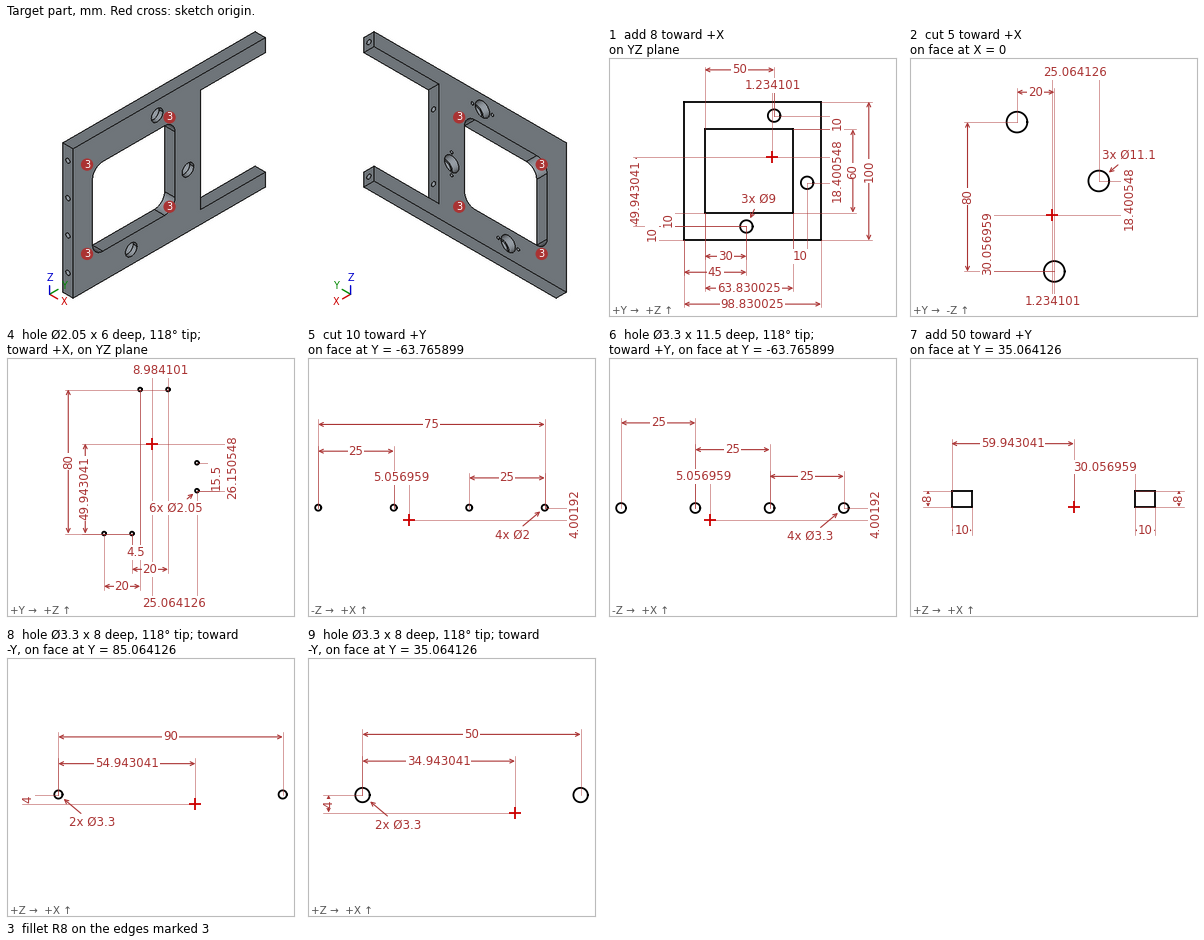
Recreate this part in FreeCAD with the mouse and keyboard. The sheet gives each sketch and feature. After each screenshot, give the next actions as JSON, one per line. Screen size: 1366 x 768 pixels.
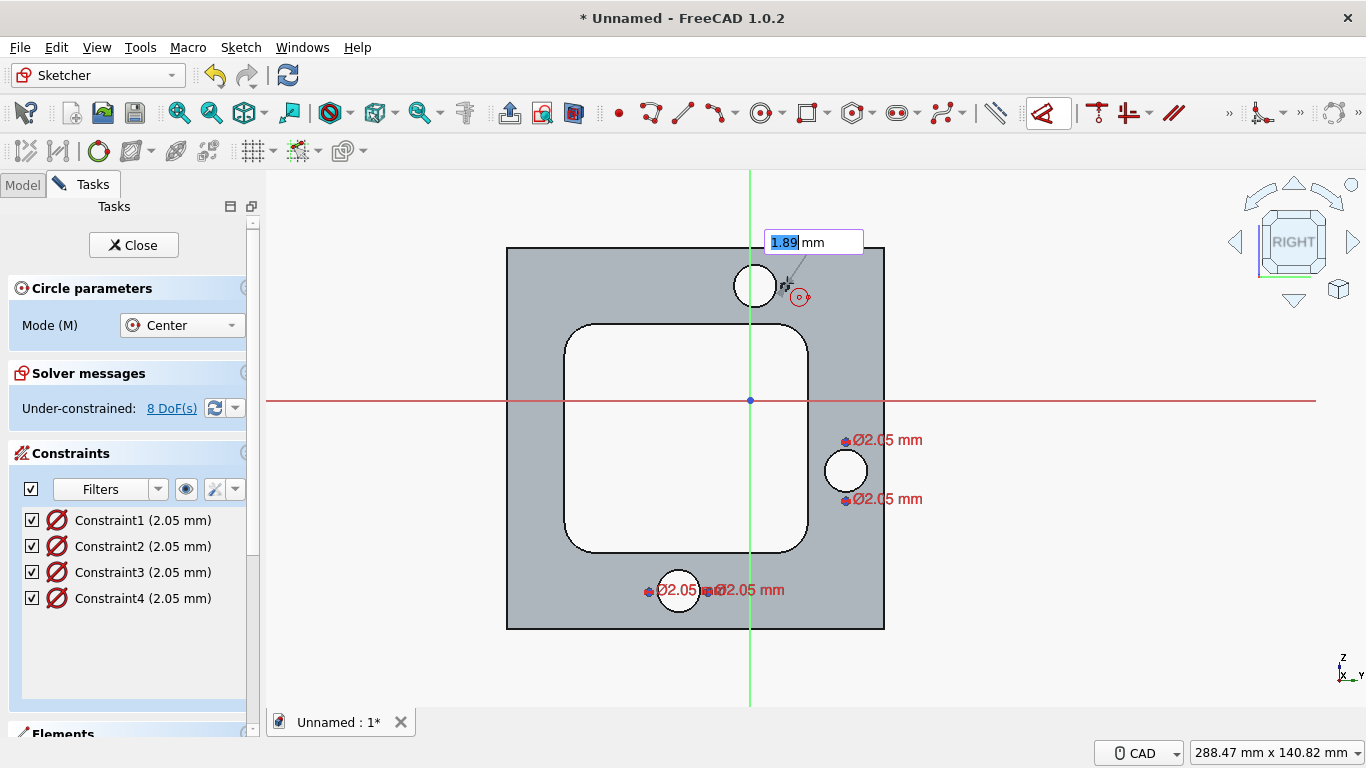
{"action": "type", "text": "2.05"}
{"action": "key", "text": "Return"}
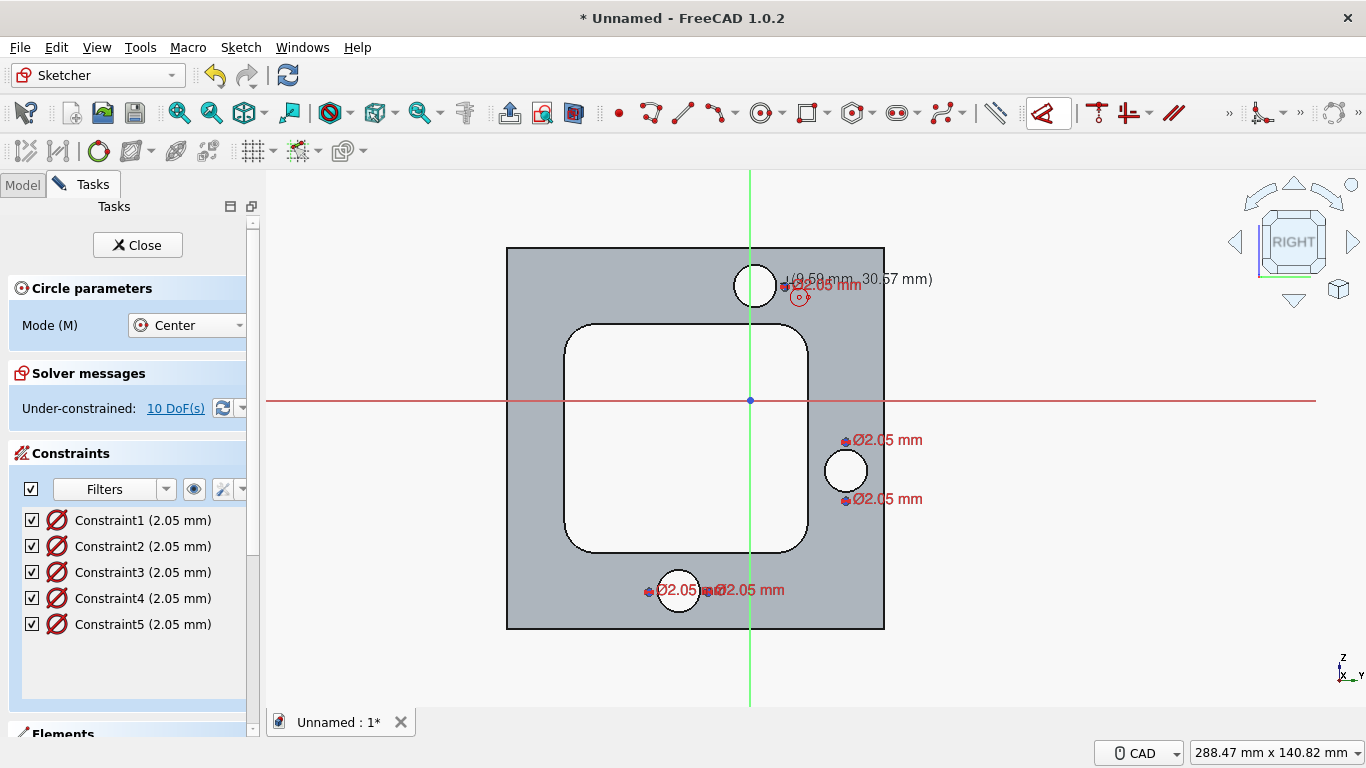
{"action": "scroll", "coordinate": [726, 286], "scroll_direction": "up", "scroll_amount": 9}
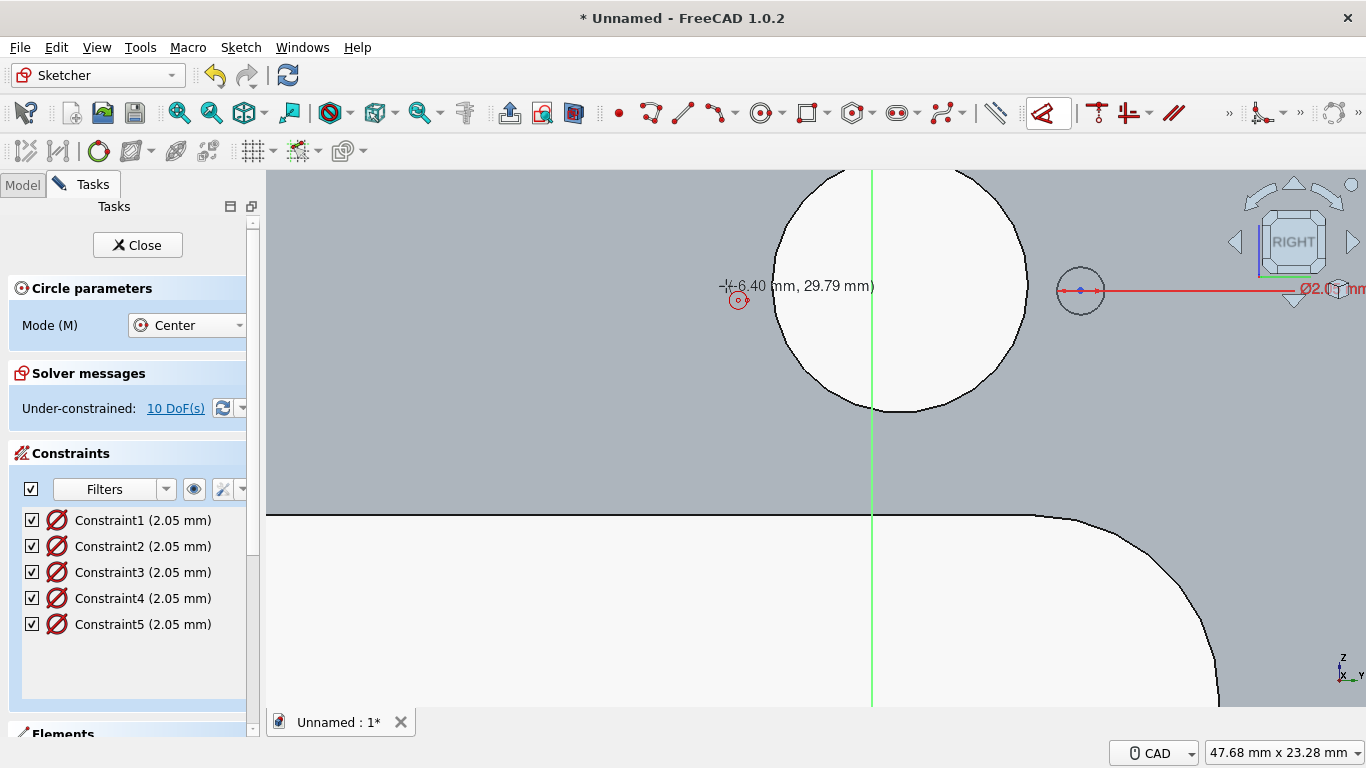
{"action": "scroll", "coordinate": [726, 286], "scroll_direction": "down", "scroll_amount": 9}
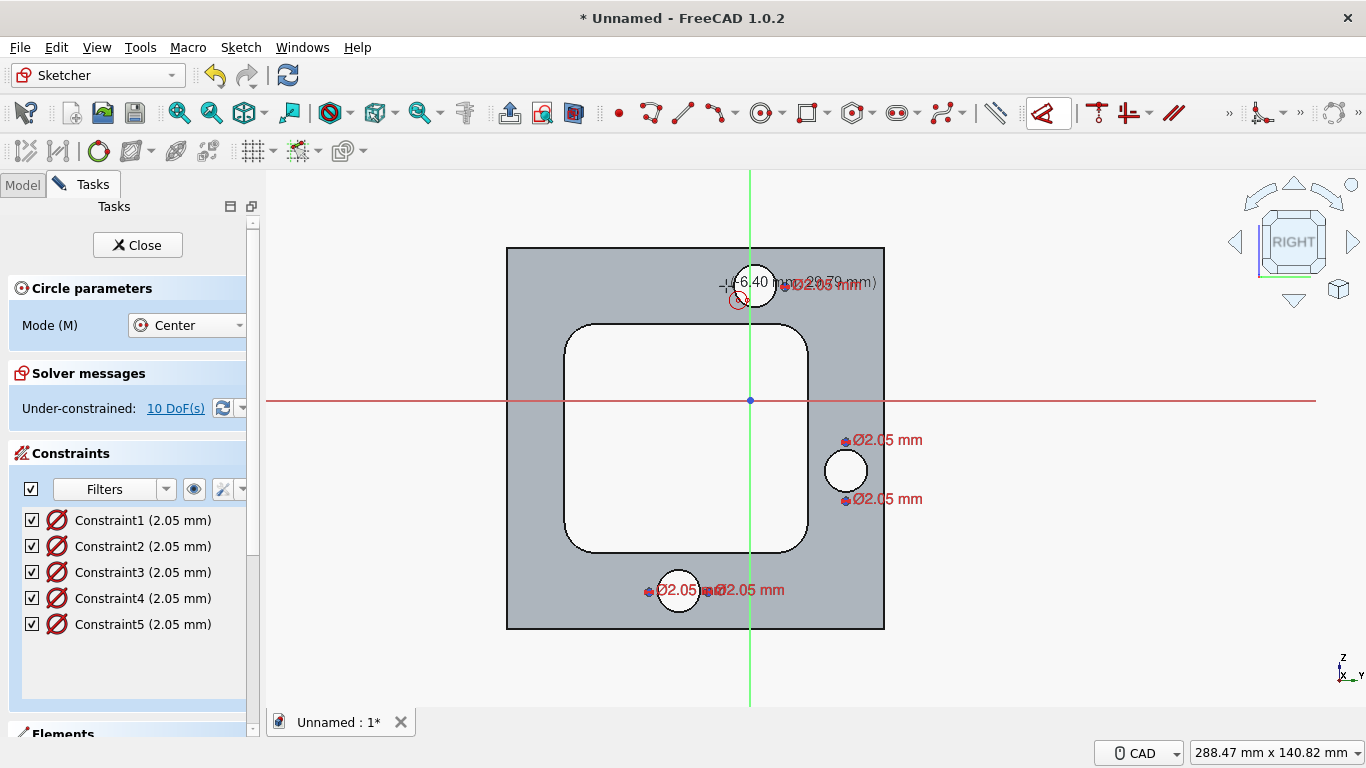
{"action": "left_click", "coordinate": [726, 286]}
{"action": "mouse_move", "coordinate": [728, 283]}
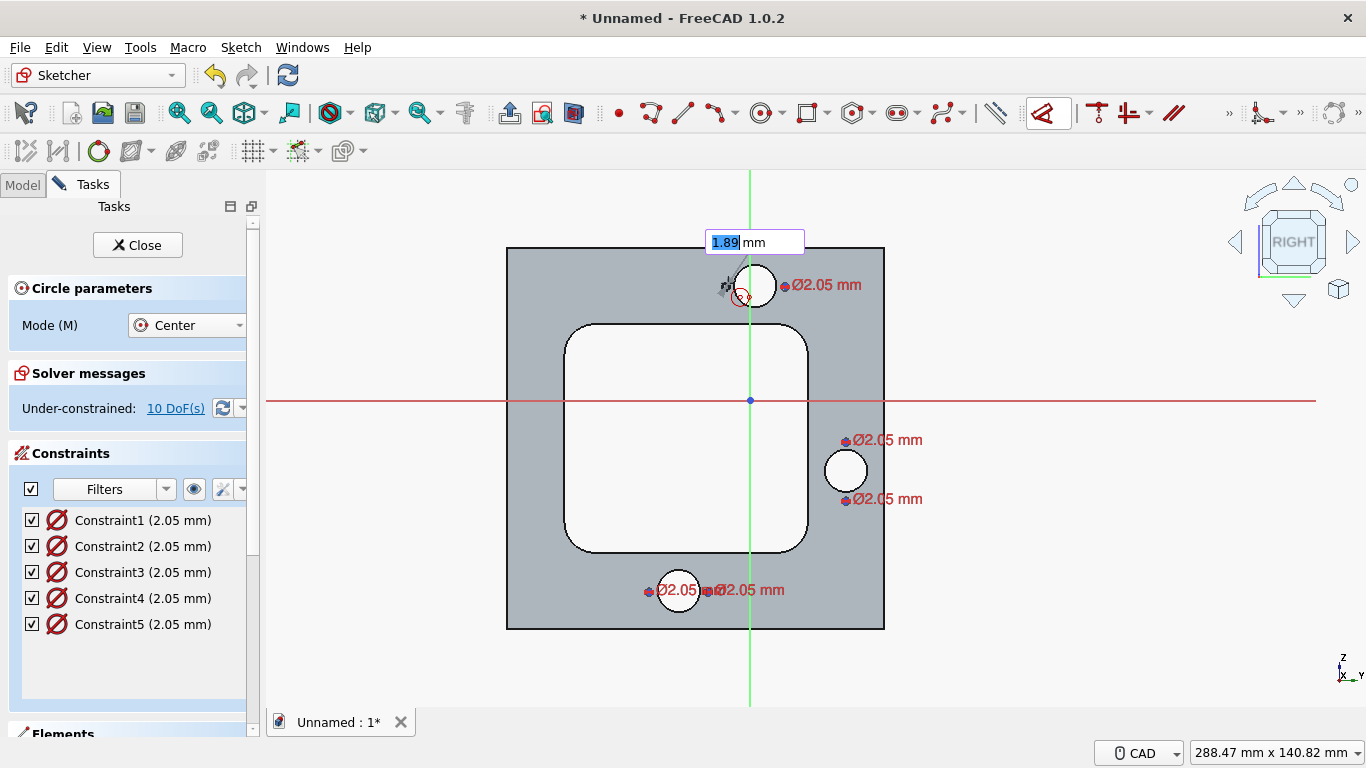
{"action": "type", "text": "2.05"}
{"action": "key", "text": "Return"}
{"action": "key", "text": "Escape"}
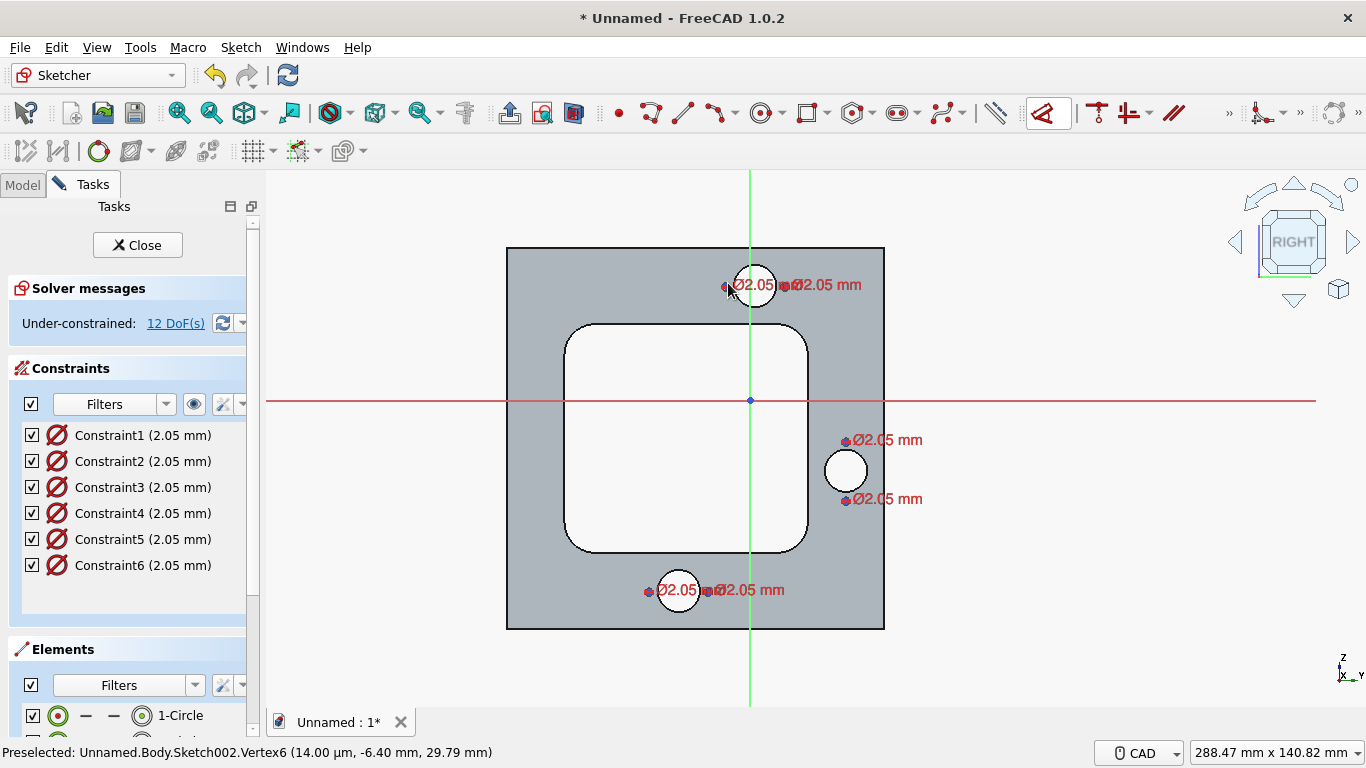
{"action": "left_click", "coordinate": [846, 501]}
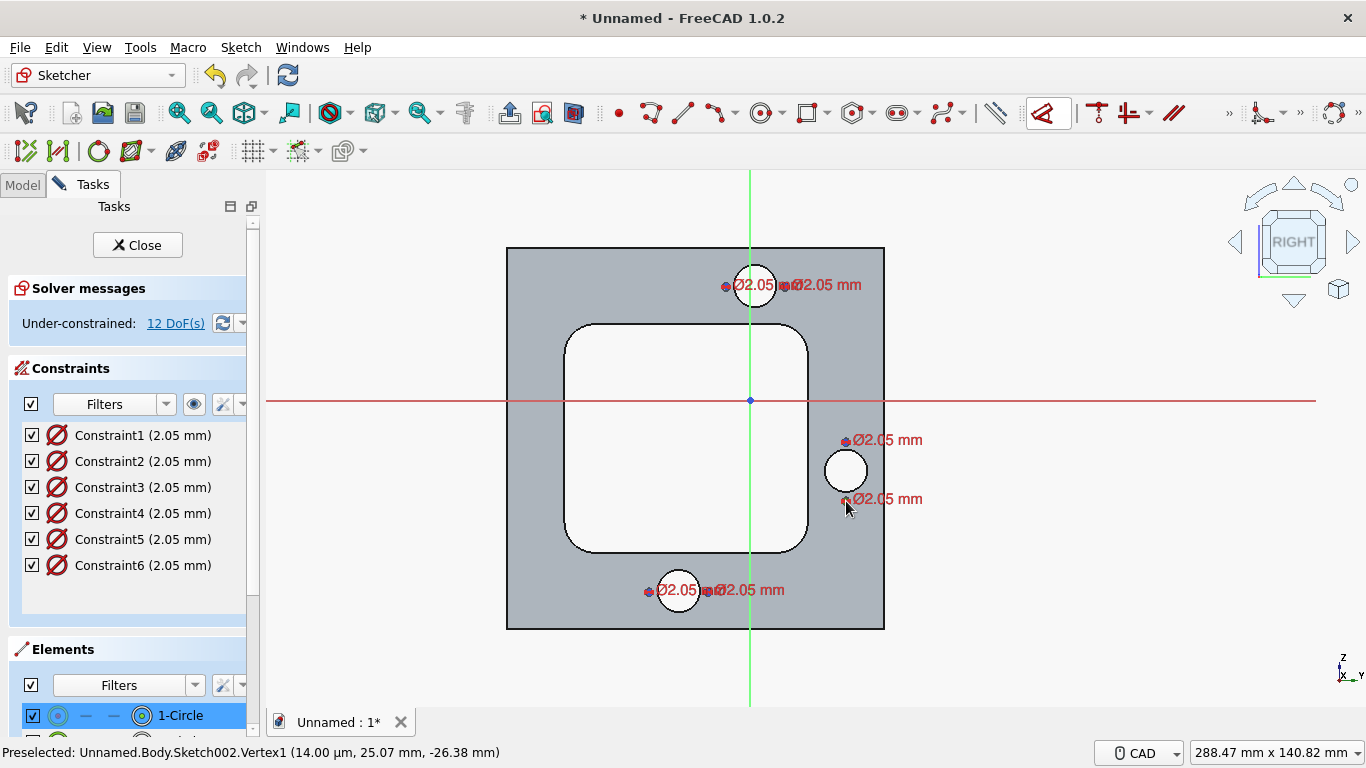
{"action": "left_click", "coordinate": [846, 442]}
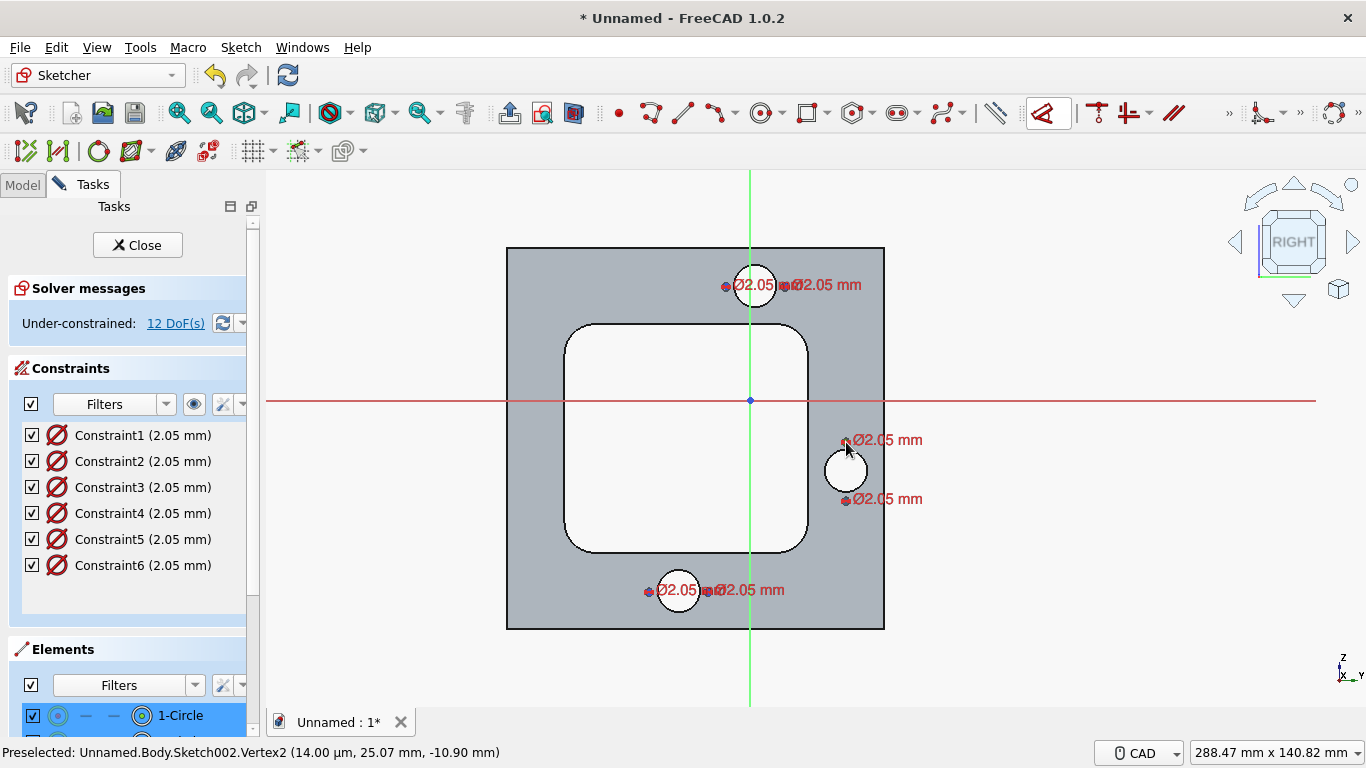
{"action": "key", "text": "v"}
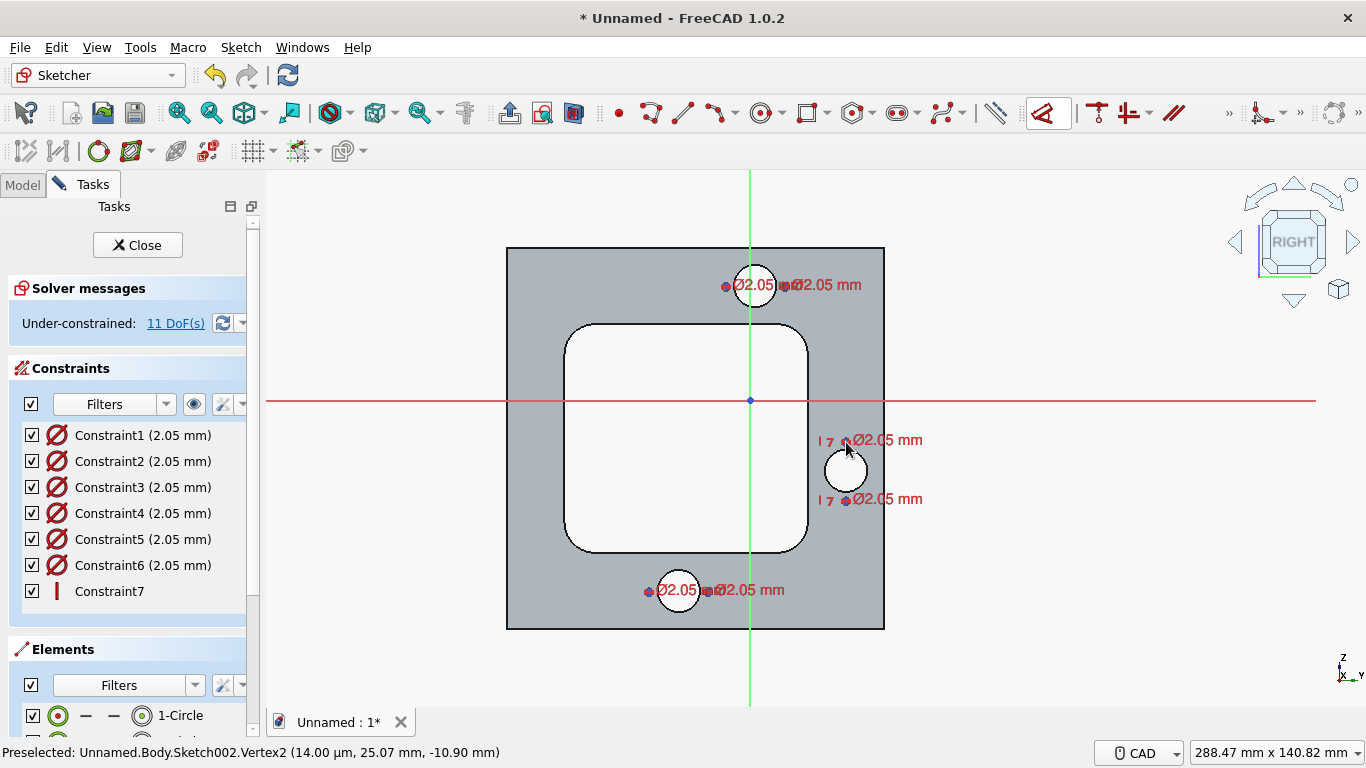
{"action": "left_click", "coordinate": [708, 592]}